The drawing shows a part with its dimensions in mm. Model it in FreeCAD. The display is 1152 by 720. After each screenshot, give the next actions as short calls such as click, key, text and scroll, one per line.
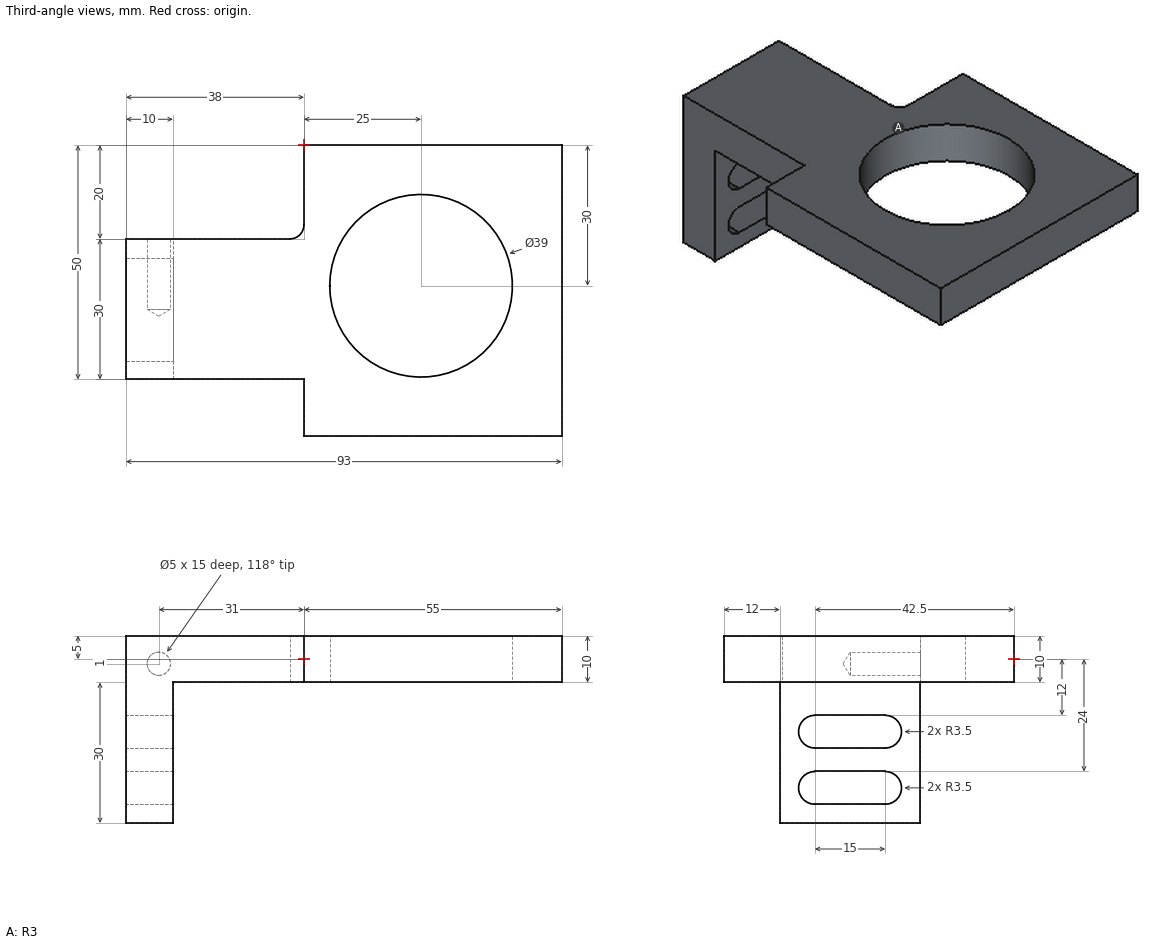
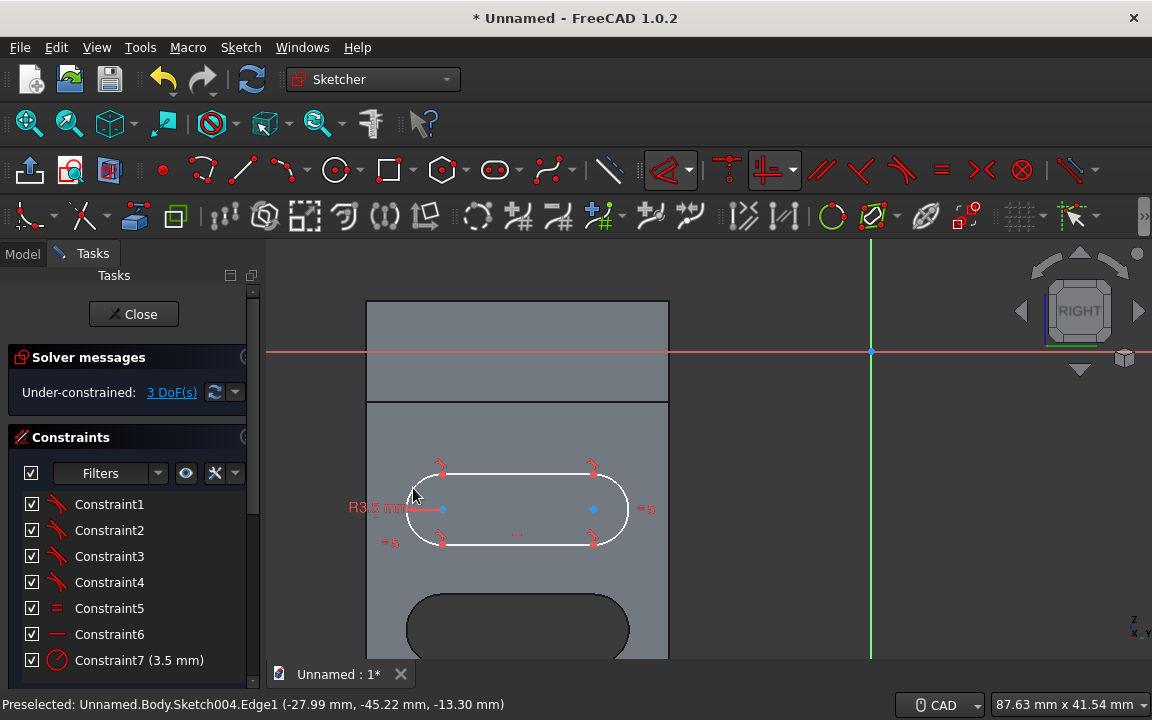
click(487, 474)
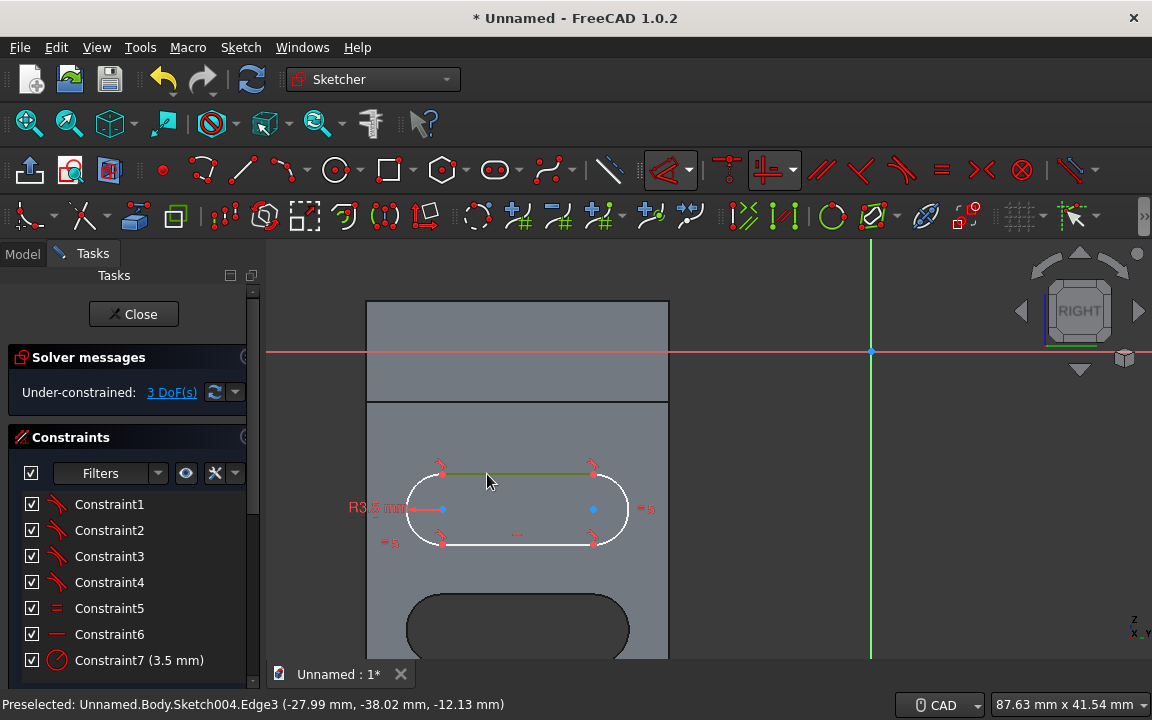
key(l)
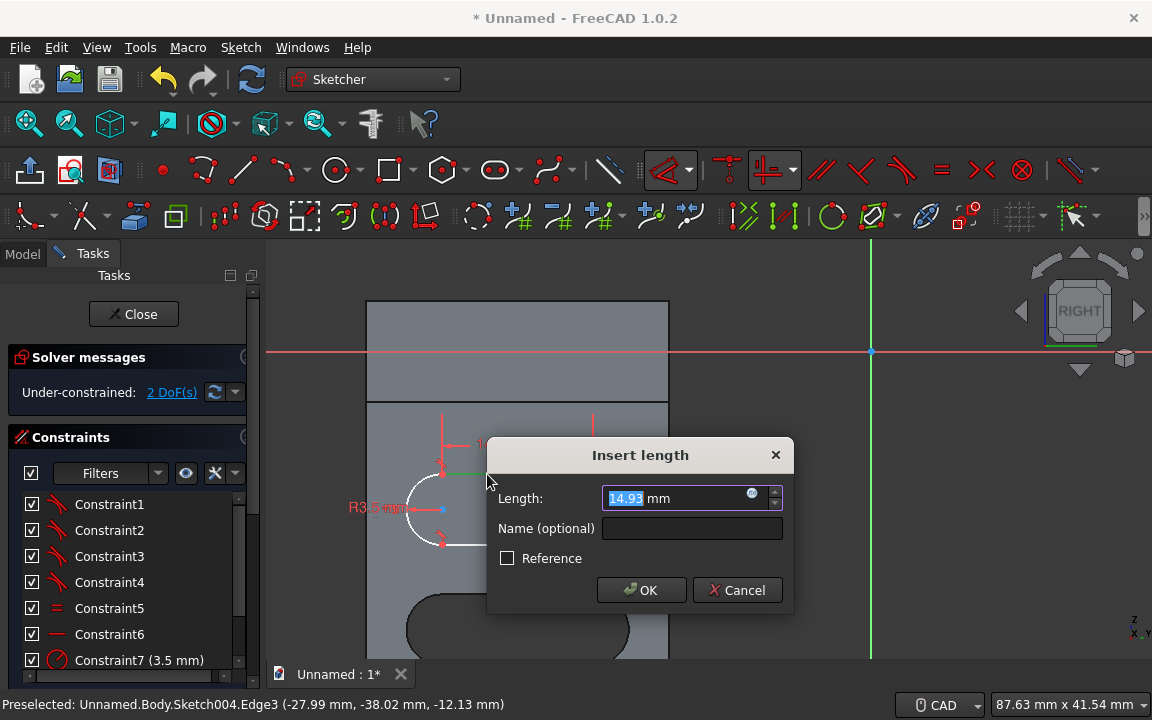
text(15)
key(Return)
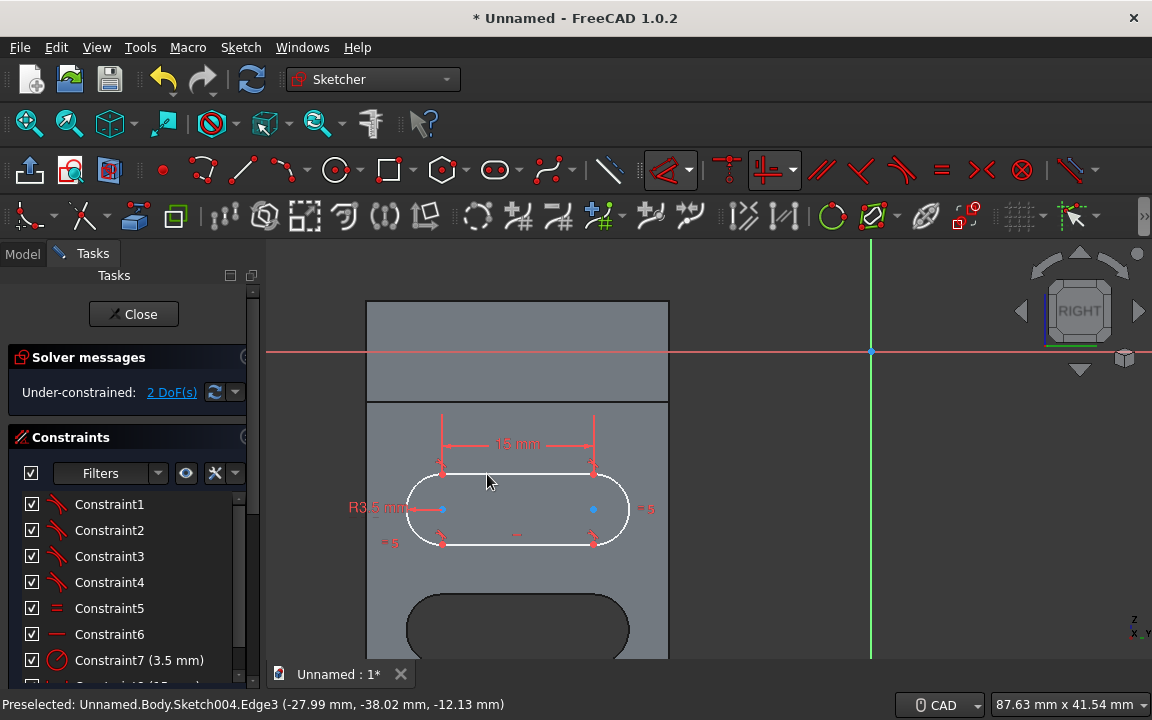
click(442, 474)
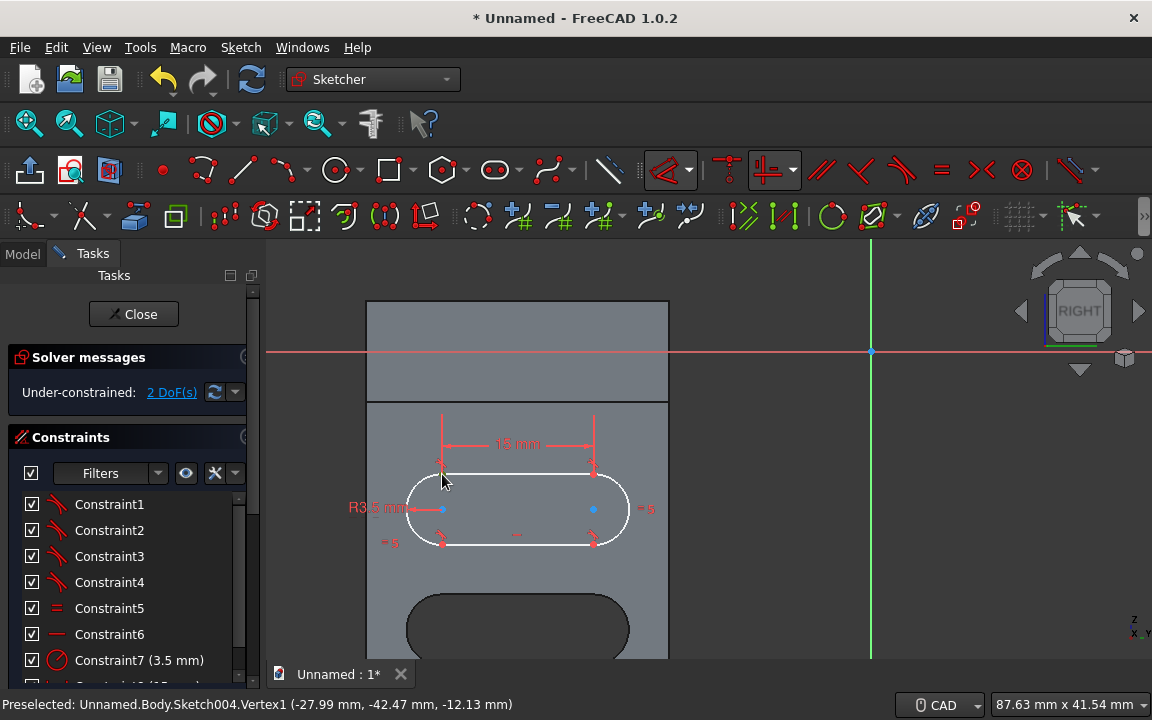
key(i)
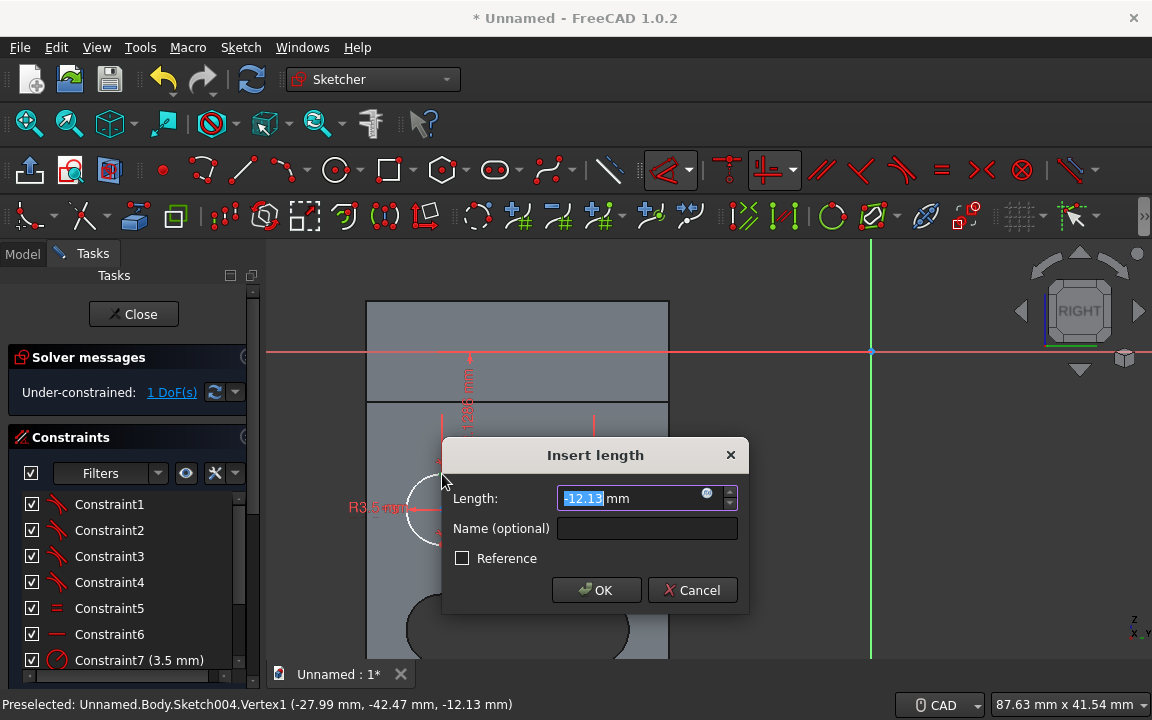
text(-12)
key(Return)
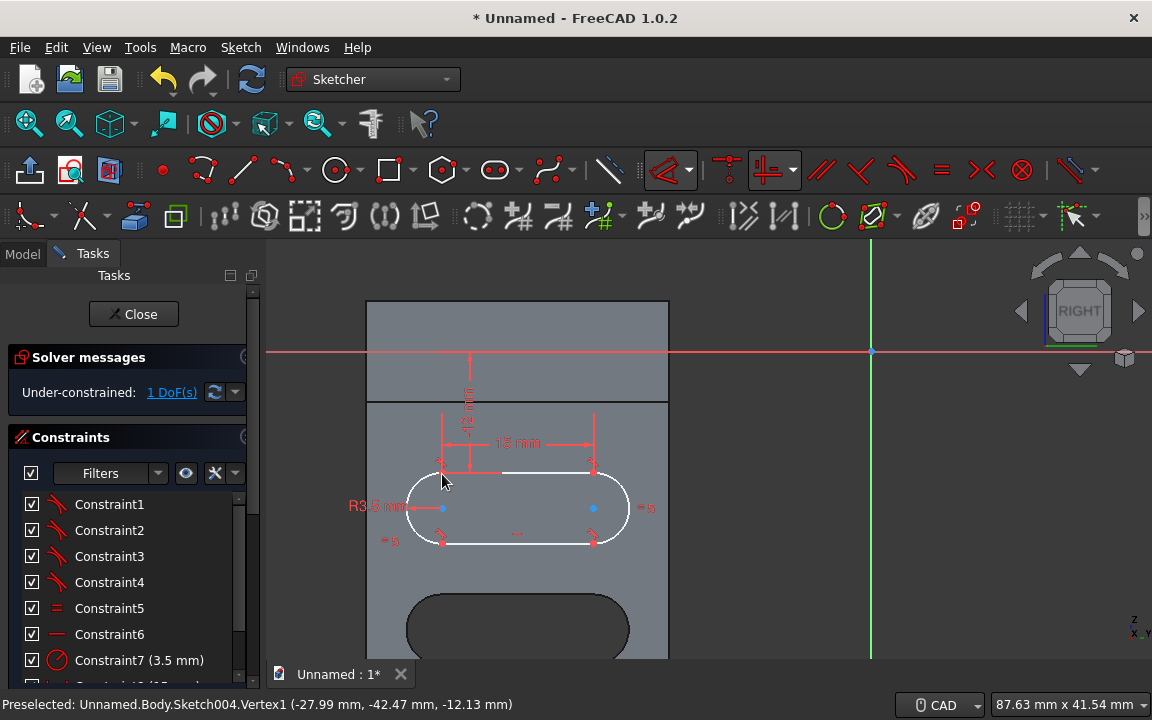
click(442, 473)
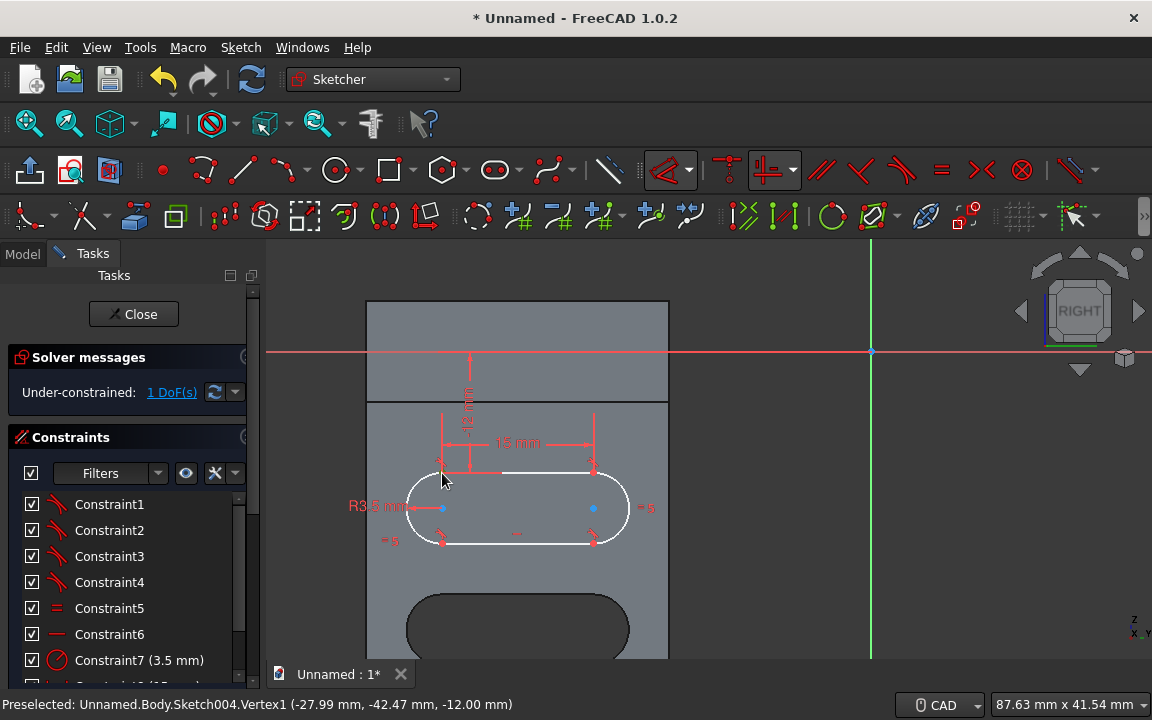
click(692, 170)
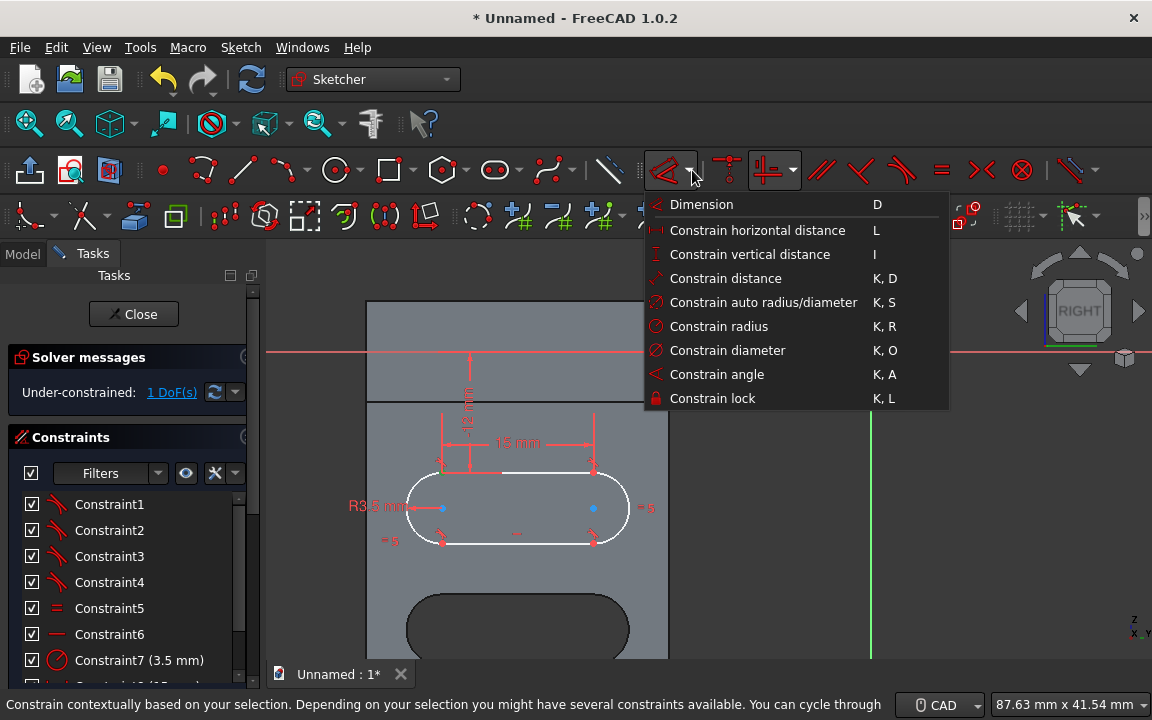
click(797, 230)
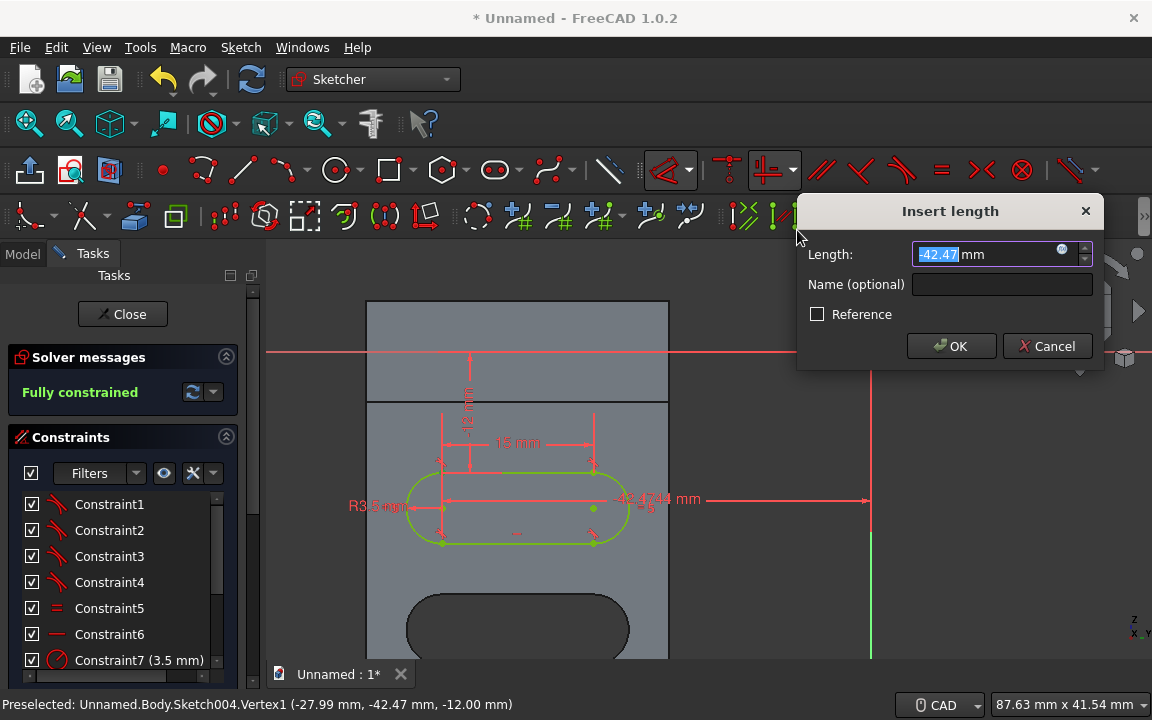
text(-42.5)
key(Return)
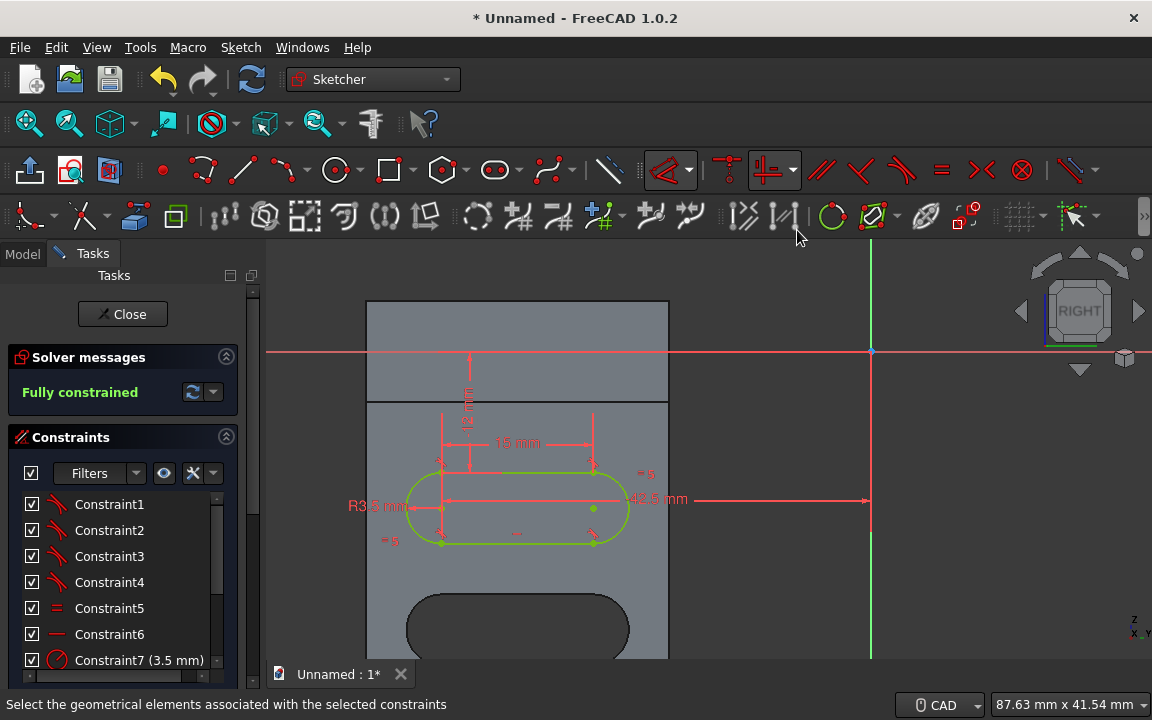
click(123, 314)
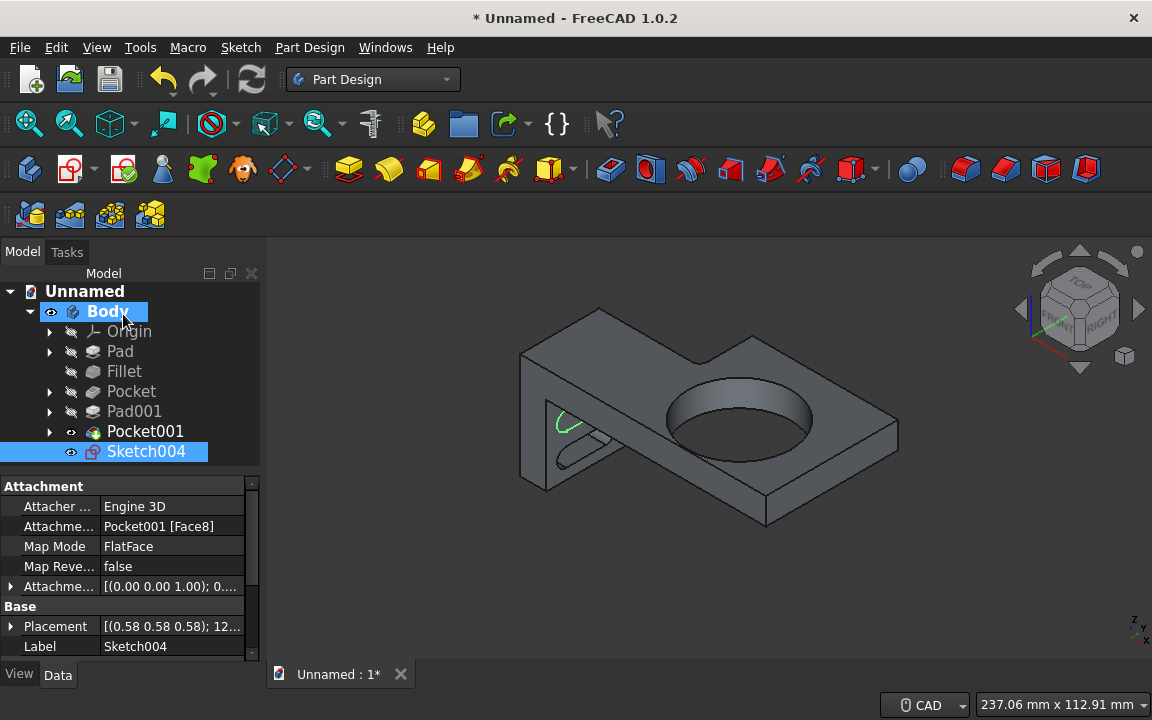
click(612, 170)